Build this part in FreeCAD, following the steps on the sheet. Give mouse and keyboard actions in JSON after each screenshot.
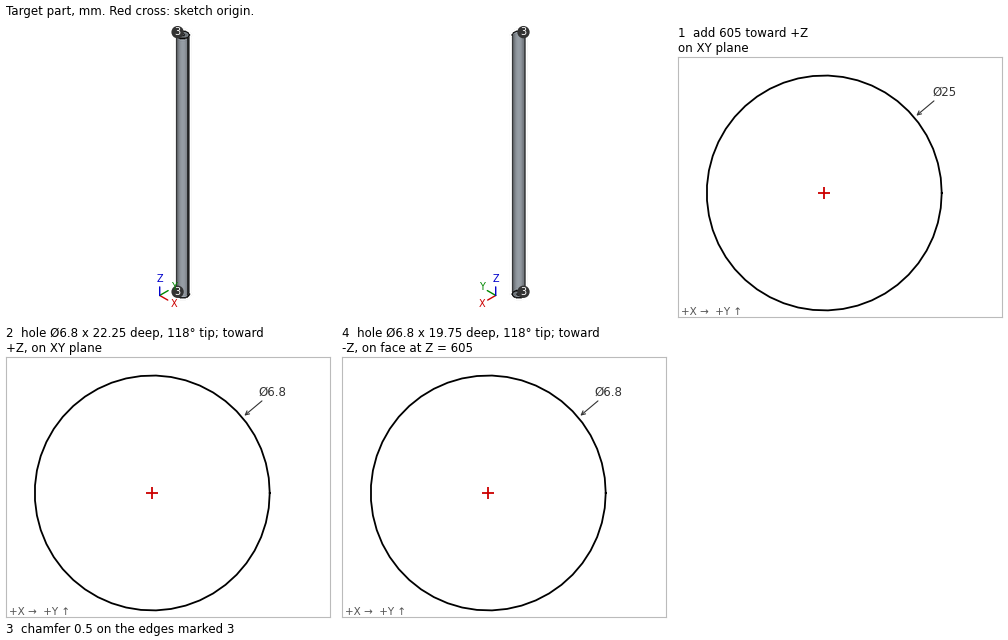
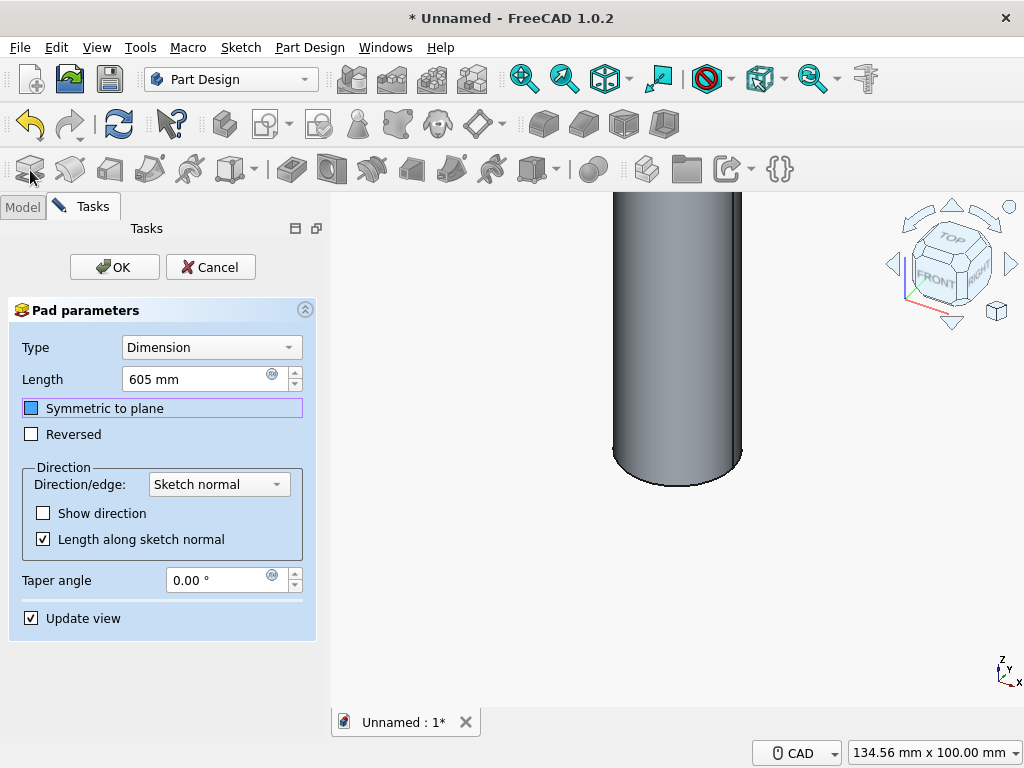
{"action": "left_click", "coordinate": [115, 267]}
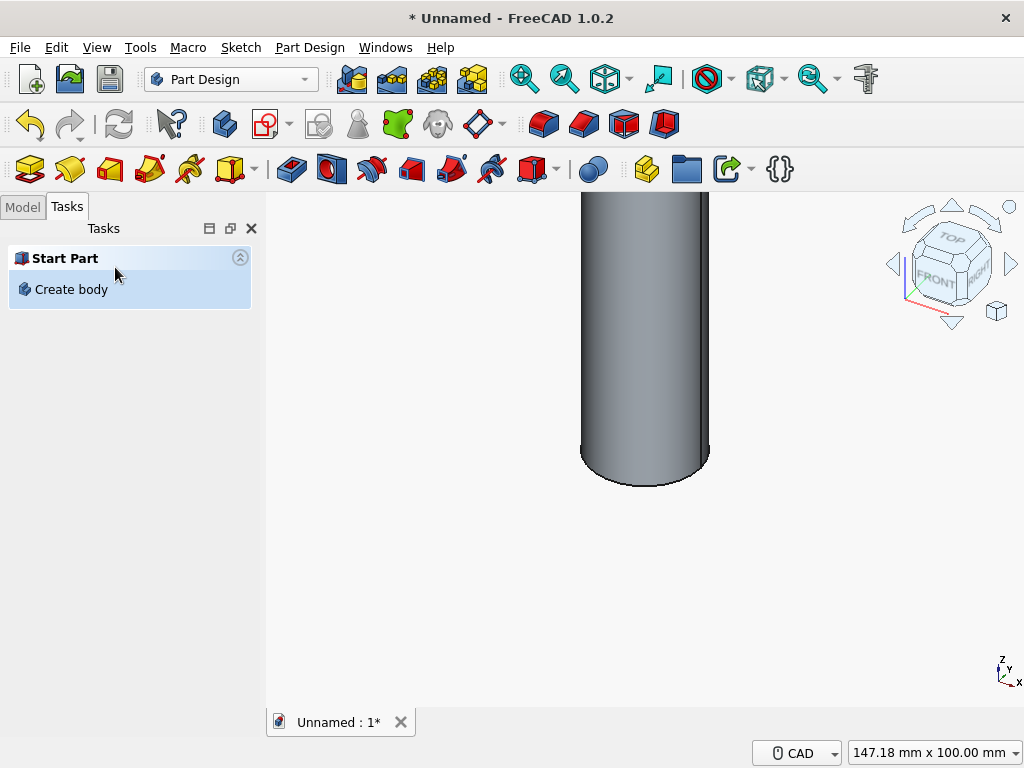
{"action": "left_click", "coordinate": [526, 80]}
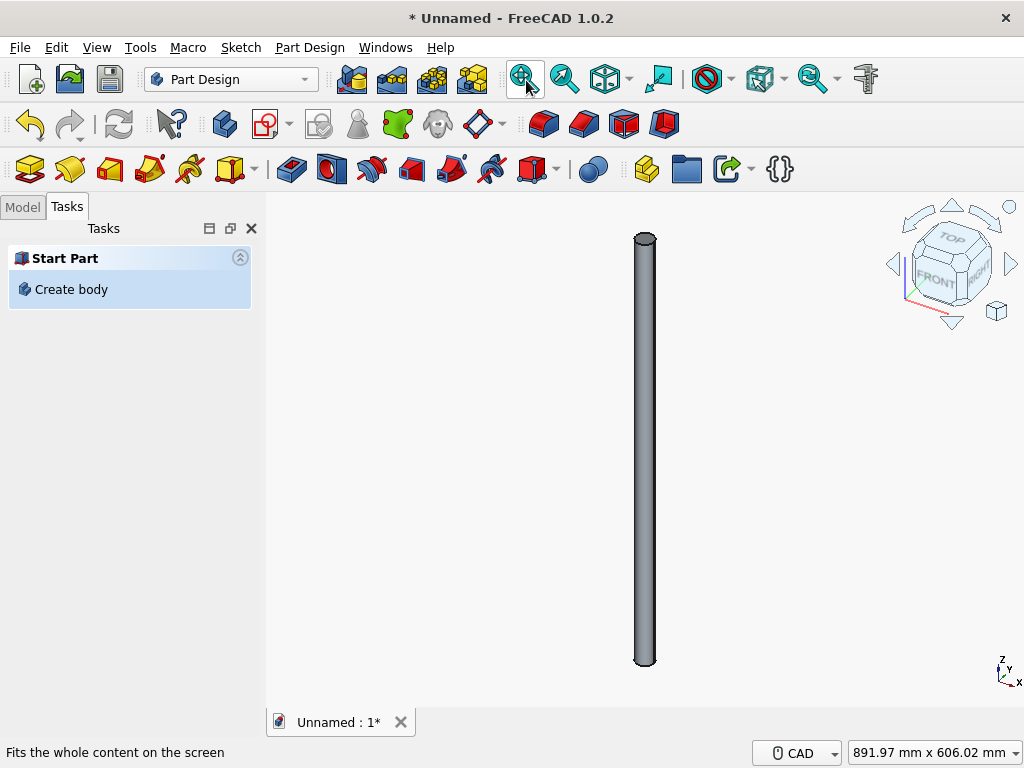
{"action": "left_click", "coordinate": [266, 124]}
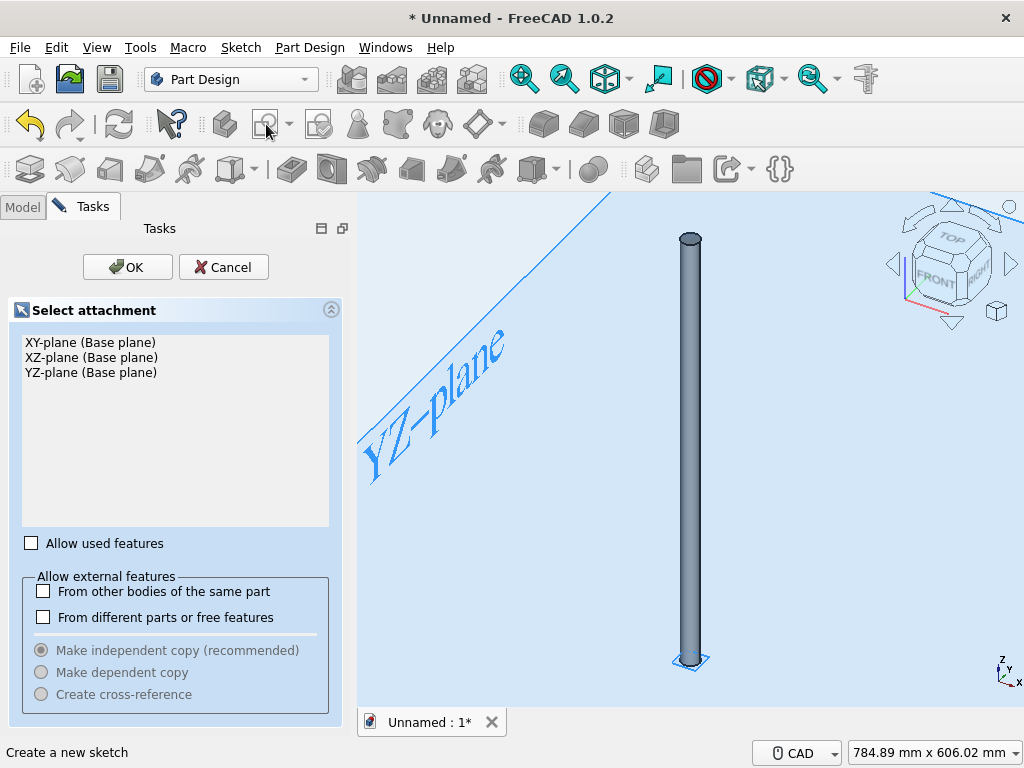
{"action": "left_click", "coordinate": [82, 342]}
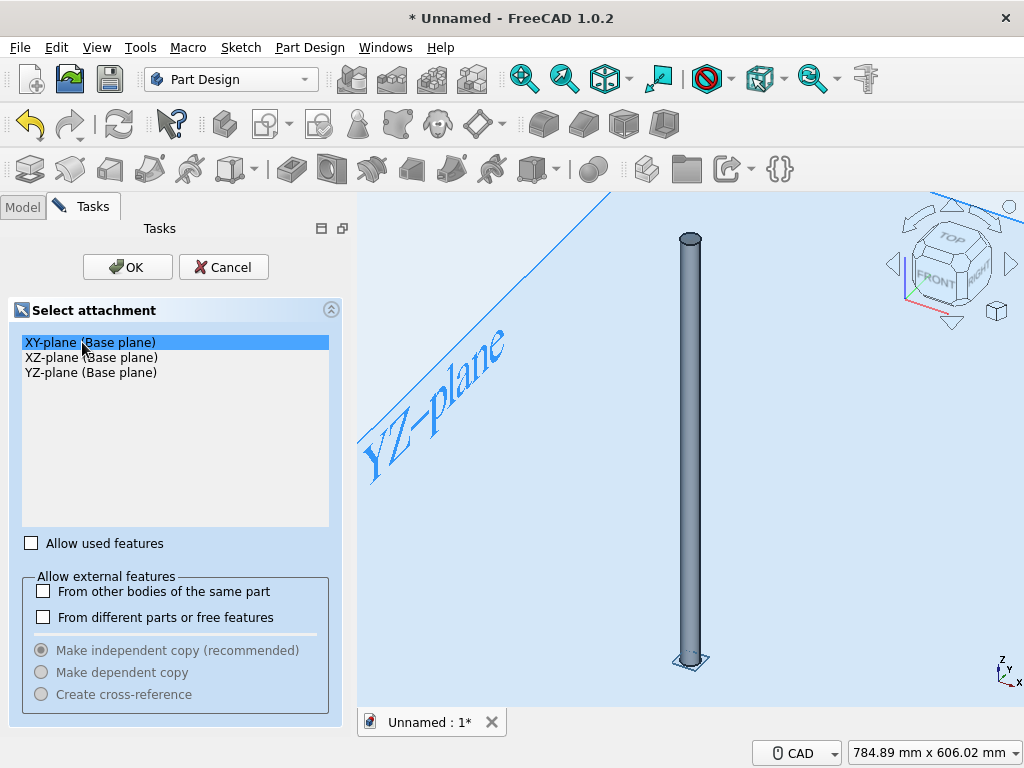
{"action": "left_click", "coordinate": [128, 267]}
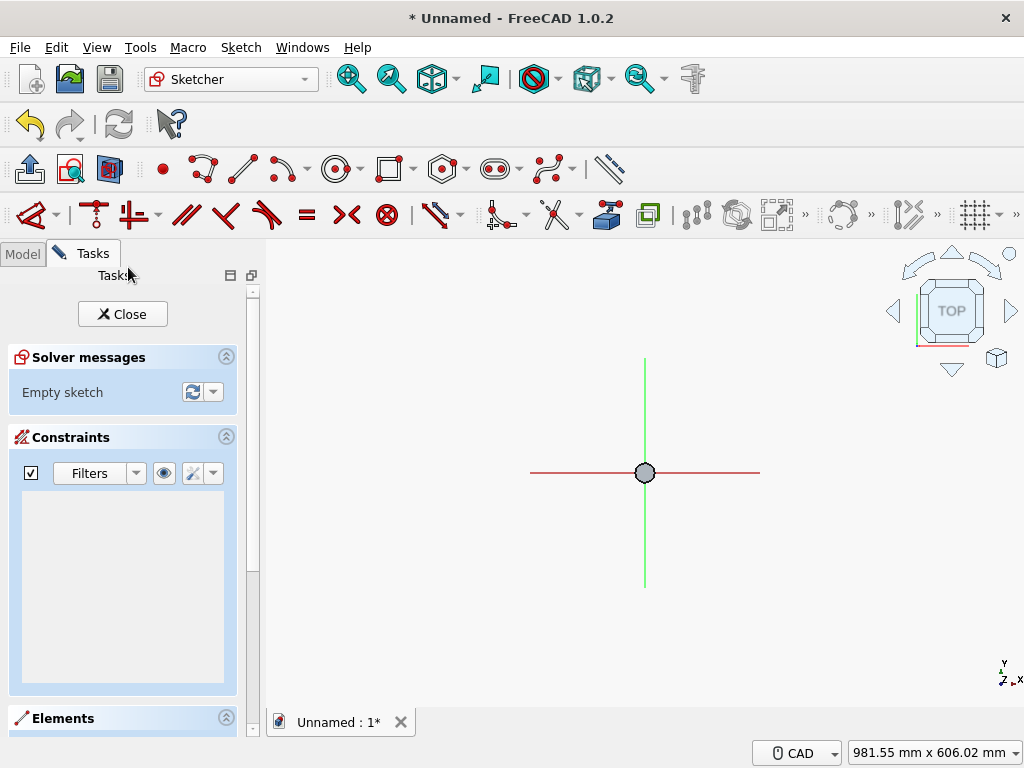
{"action": "left_click", "coordinate": [110, 170]}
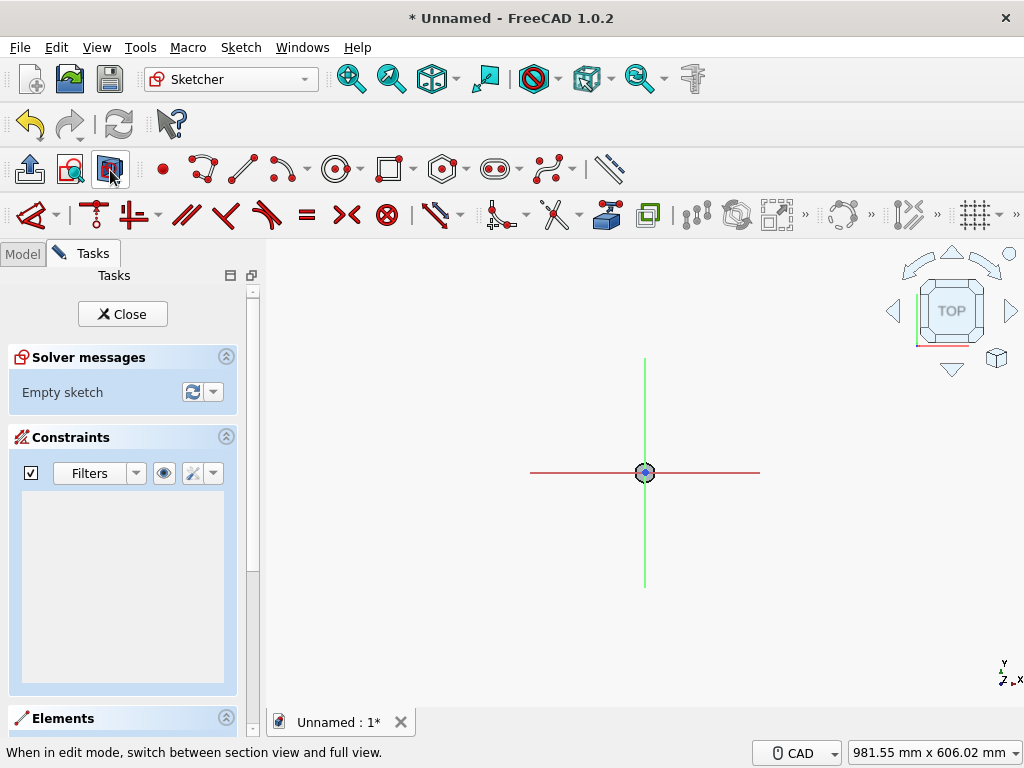
{"action": "scroll", "coordinate": [649, 473], "scroll_direction": "up", "scroll_amount": 15}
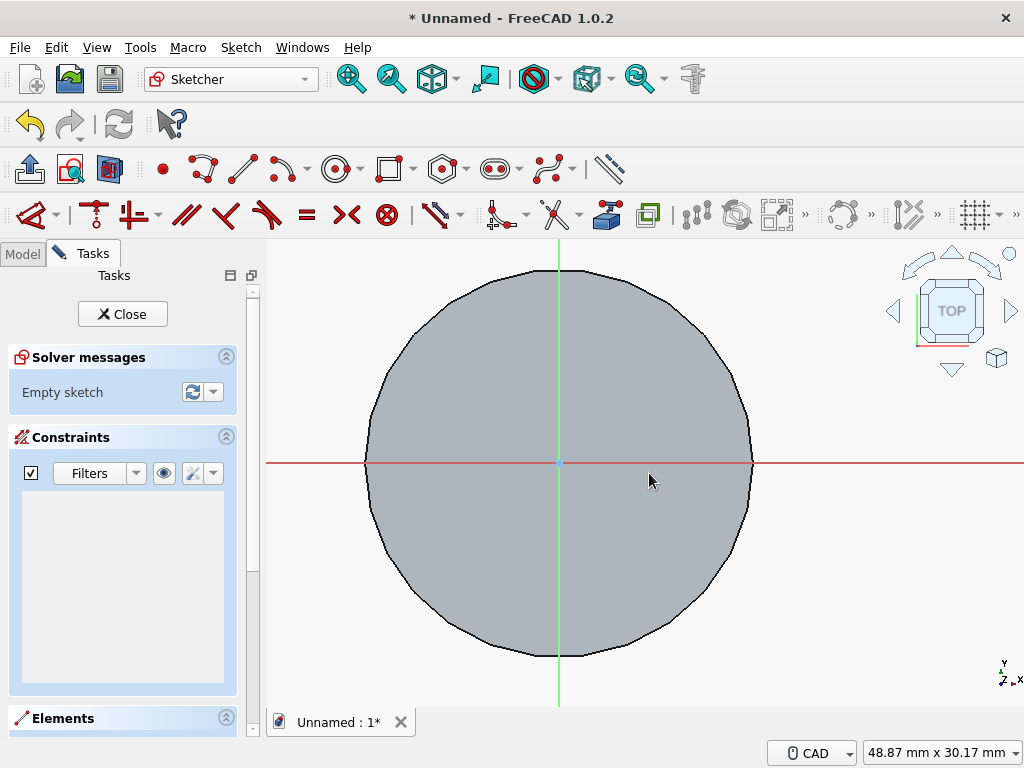
{"action": "scroll", "coordinate": [549, 458], "scroll_direction": "up", "scroll_amount": 5}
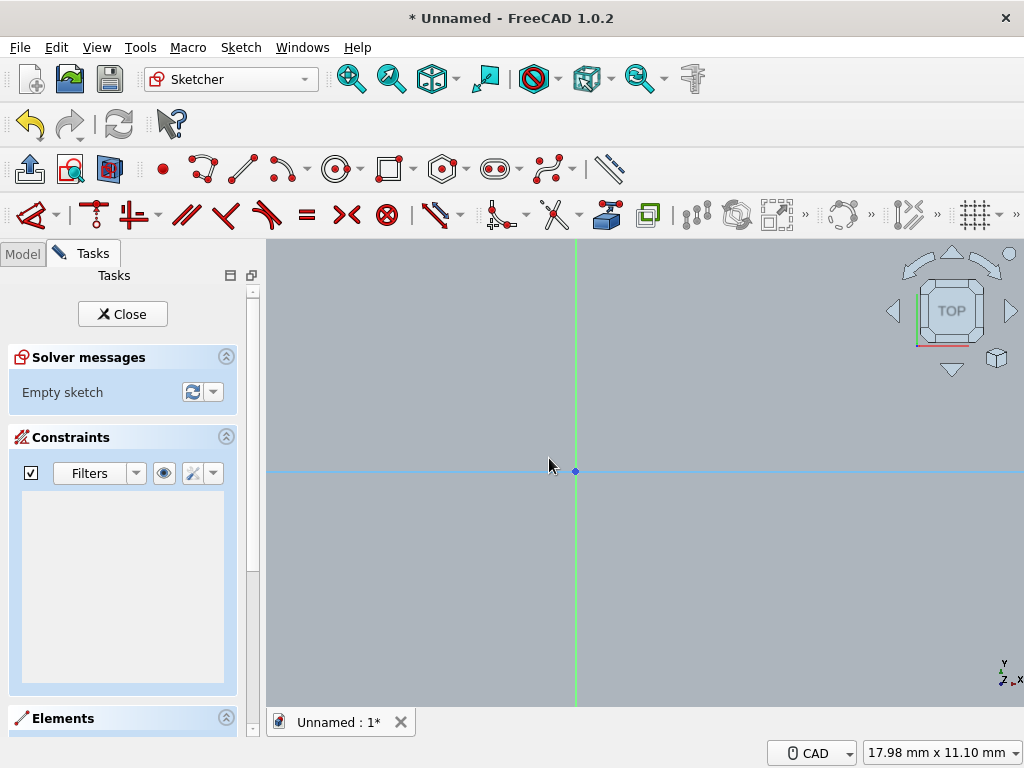
{"action": "left_click", "coordinate": [336, 170]}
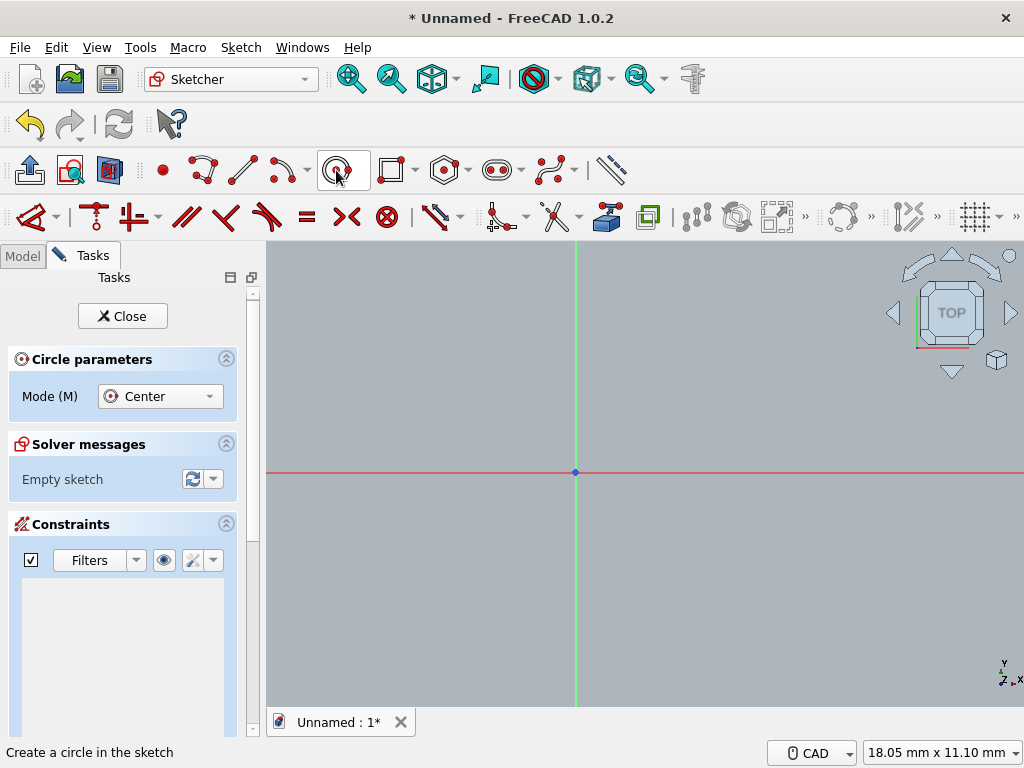
{"action": "left_click", "coordinate": [576, 473]}
{"action": "left_click", "coordinate": [677, 372]}
{"action": "key", "text": "Escape"}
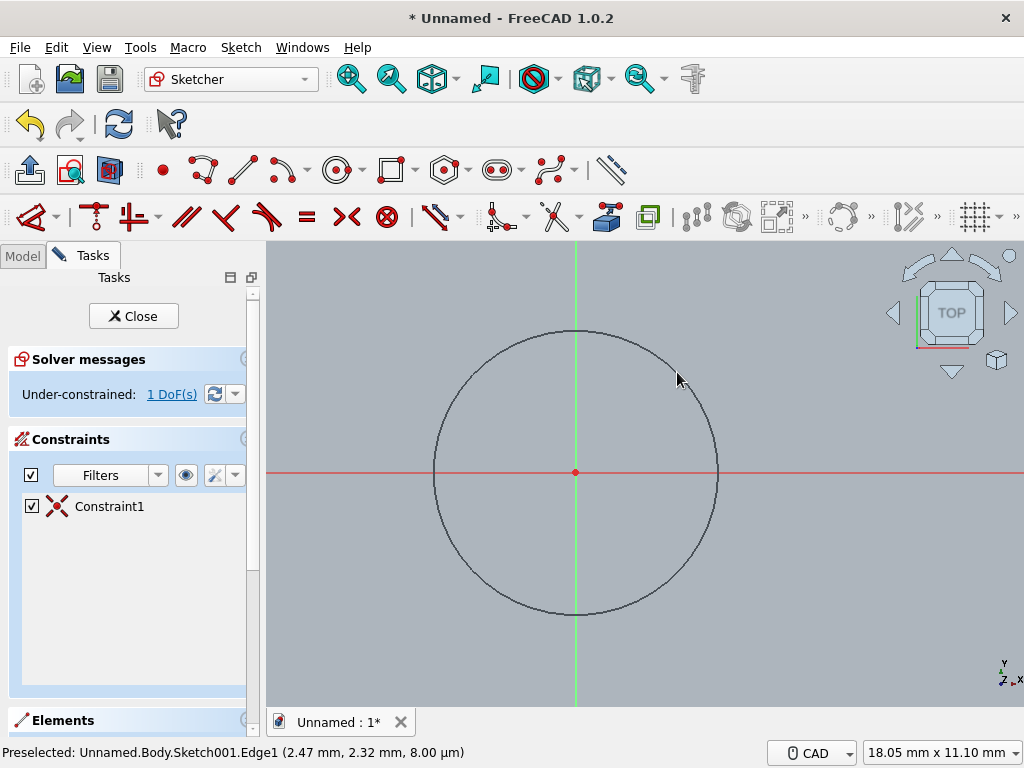
{"action": "left_click", "coordinate": [32, 218]}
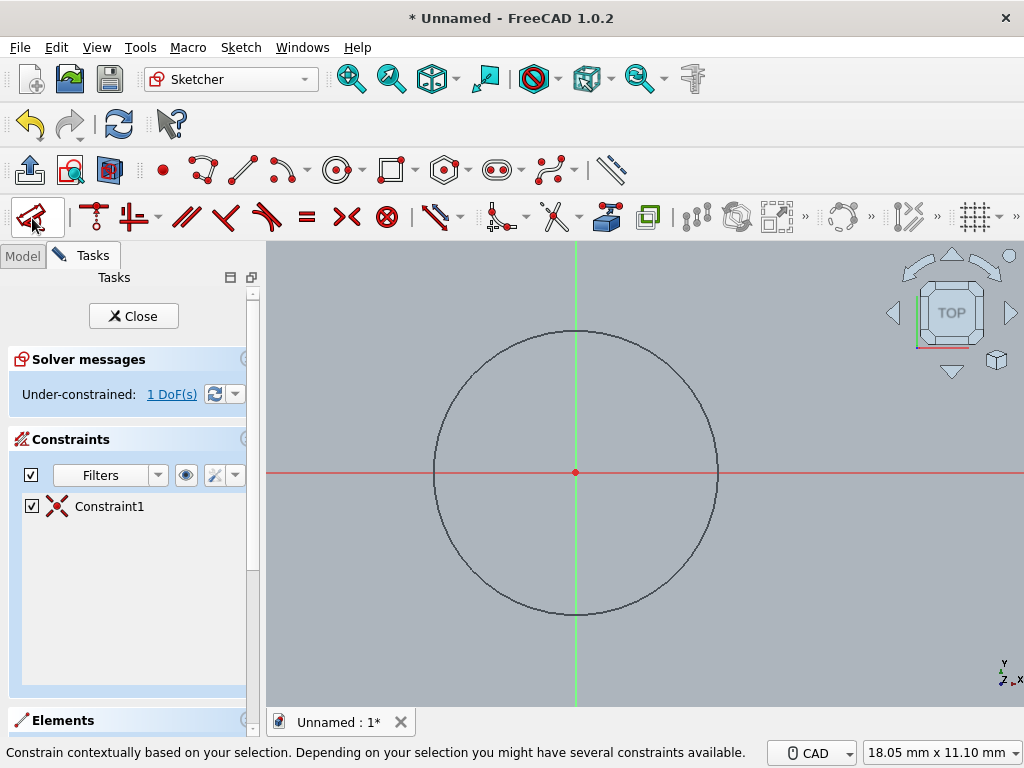
{"action": "left_click", "coordinate": [676, 372]}
{"action": "left_click", "coordinate": [699, 349]}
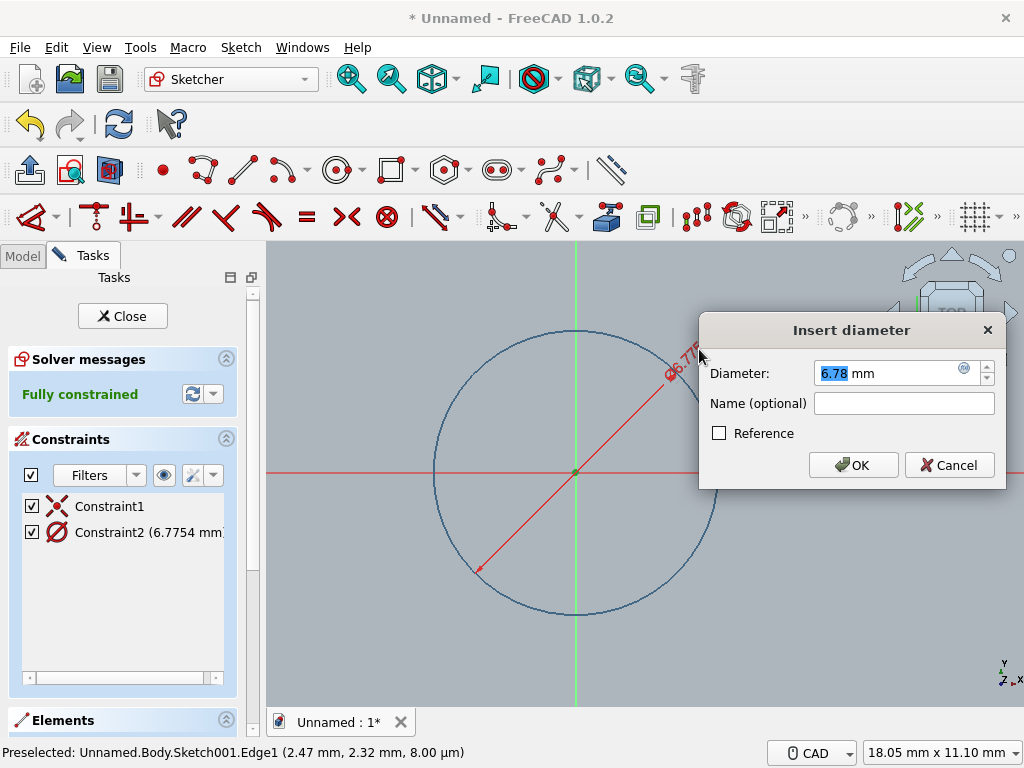
{"action": "type", "text": "6.8"}
{"action": "key", "text": "Return"}
{"action": "key", "text": "Escape"}